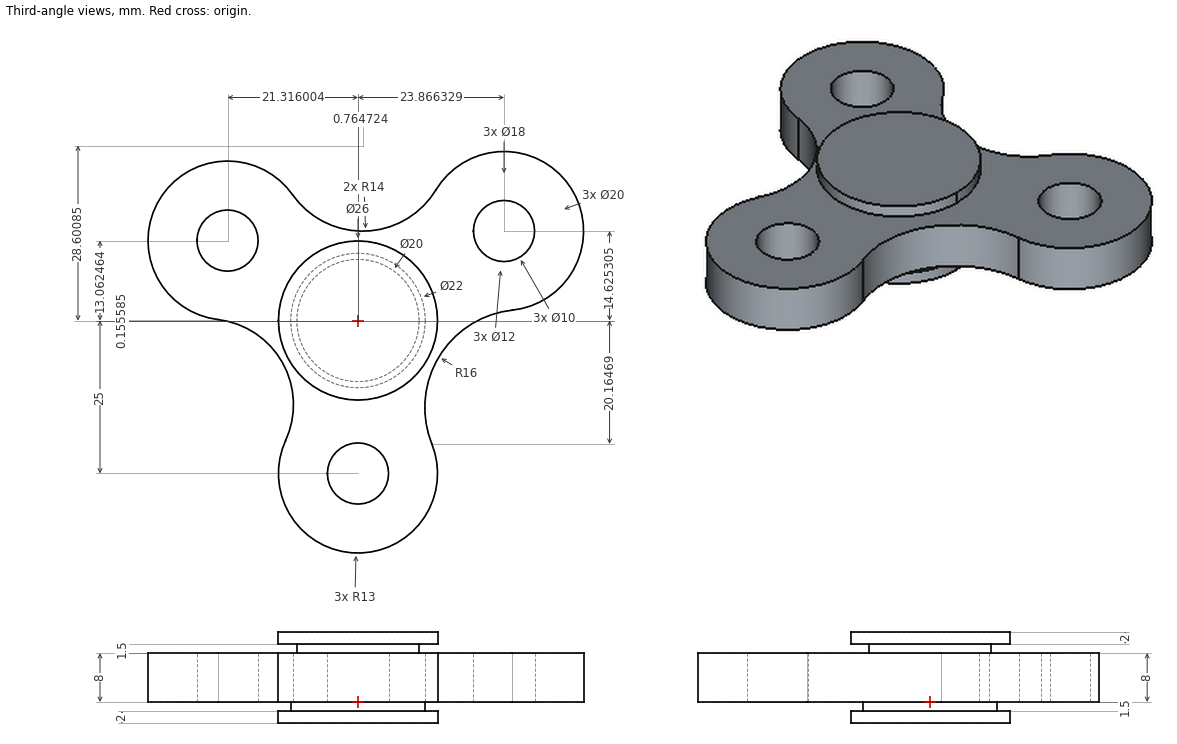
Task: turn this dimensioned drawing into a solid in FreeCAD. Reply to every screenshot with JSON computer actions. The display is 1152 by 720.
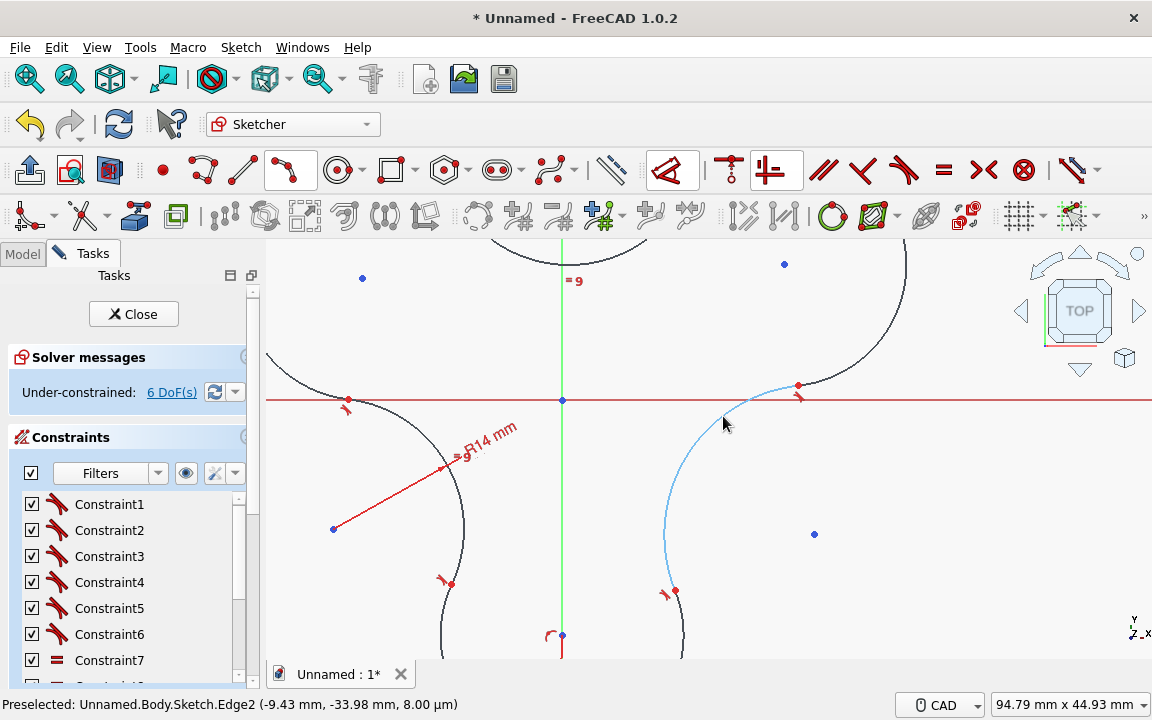
{"action": "left_click", "coordinate": [722, 416]}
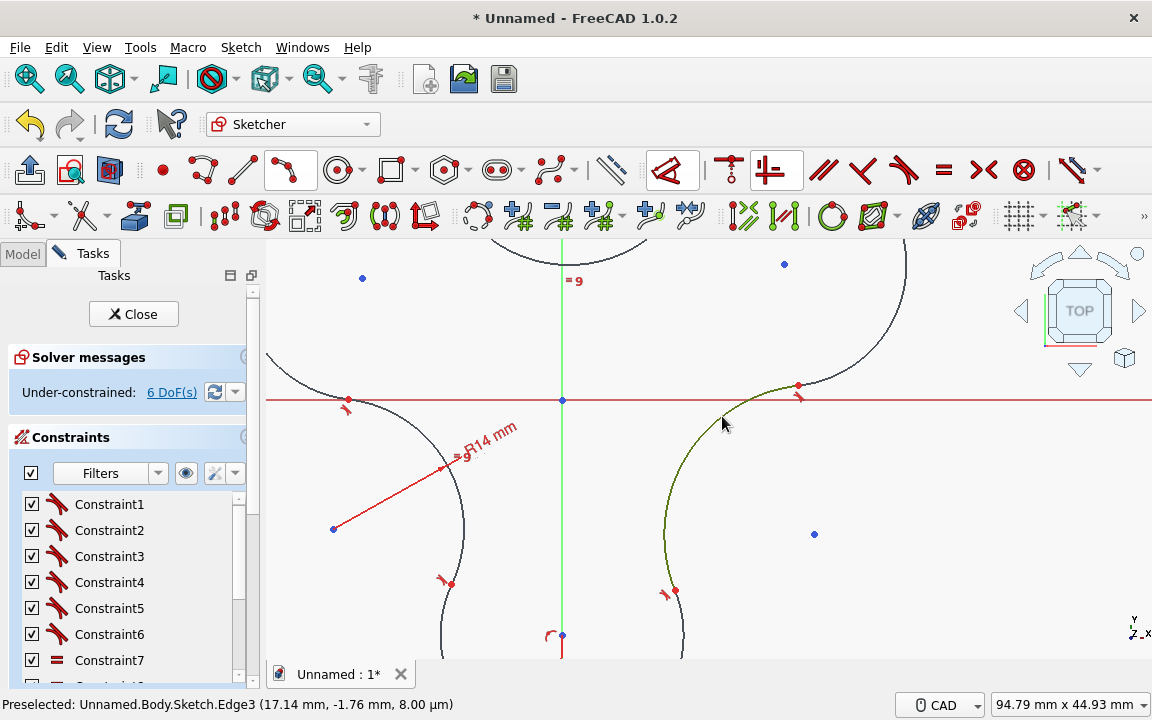
{"action": "left_click", "coordinate": [694, 170]}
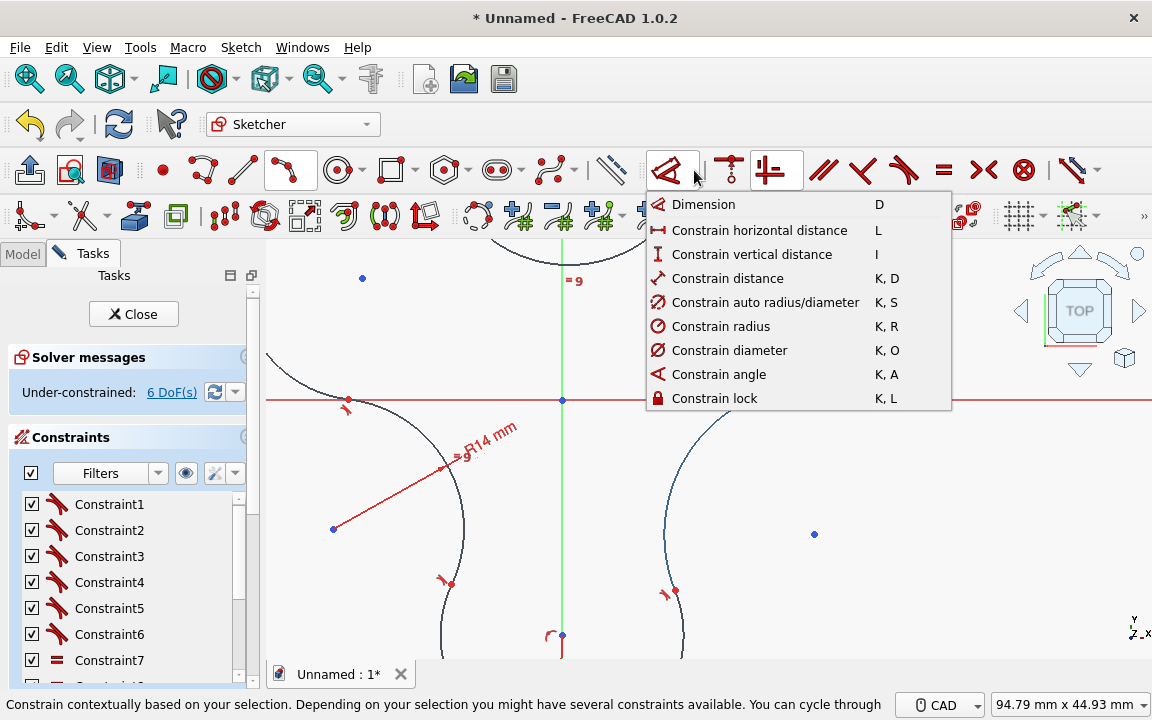
{"action": "left_click", "coordinate": [799, 326]}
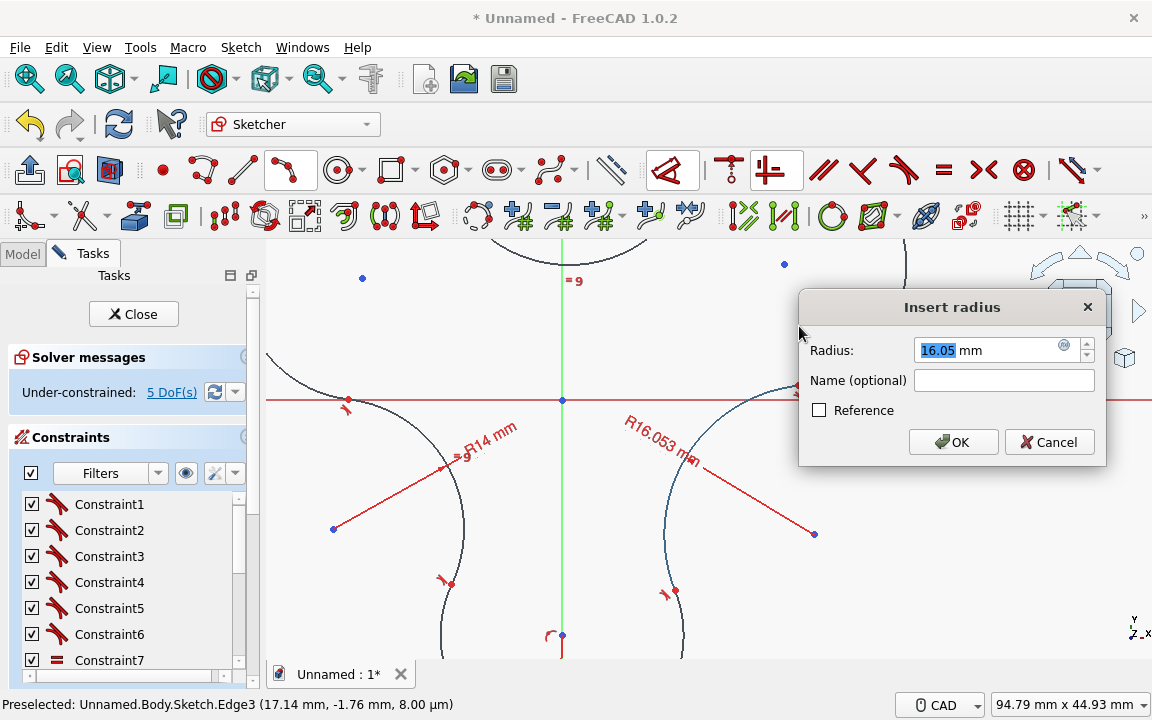
{"action": "type", "text": "16"}
{"action": "key", "text": "Return"}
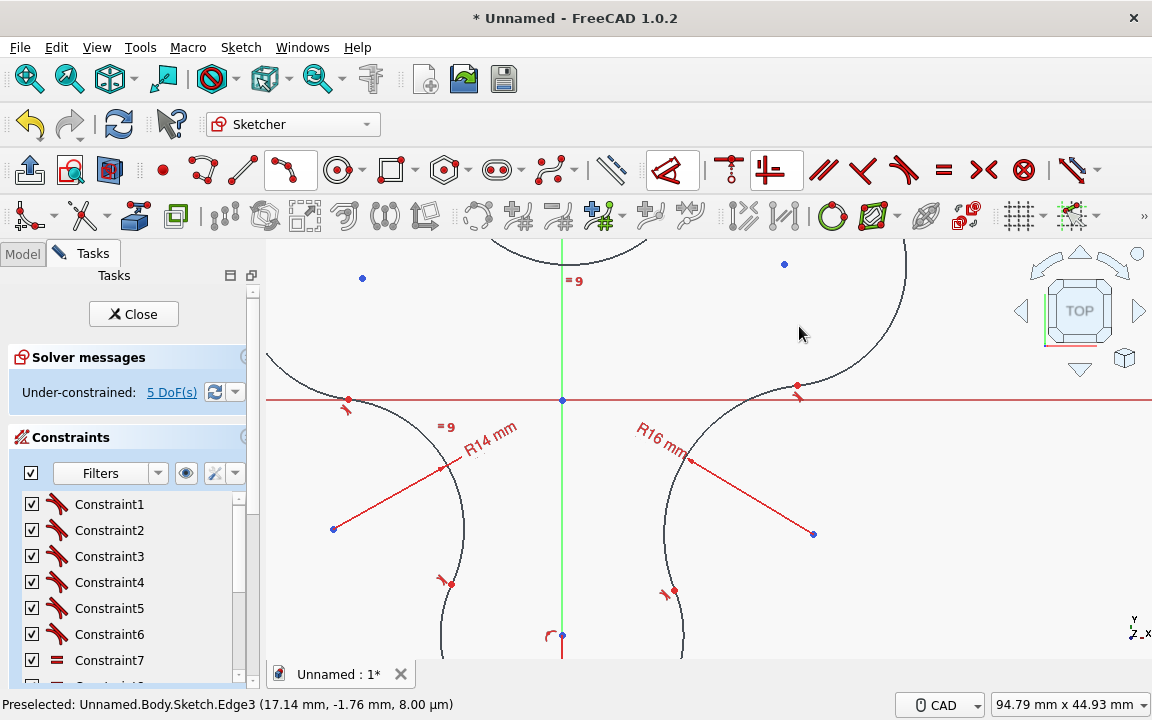
{"action": "scroll", "coordinate": [695, 426], "scroll_direction": "down", "scroll_amount": 4}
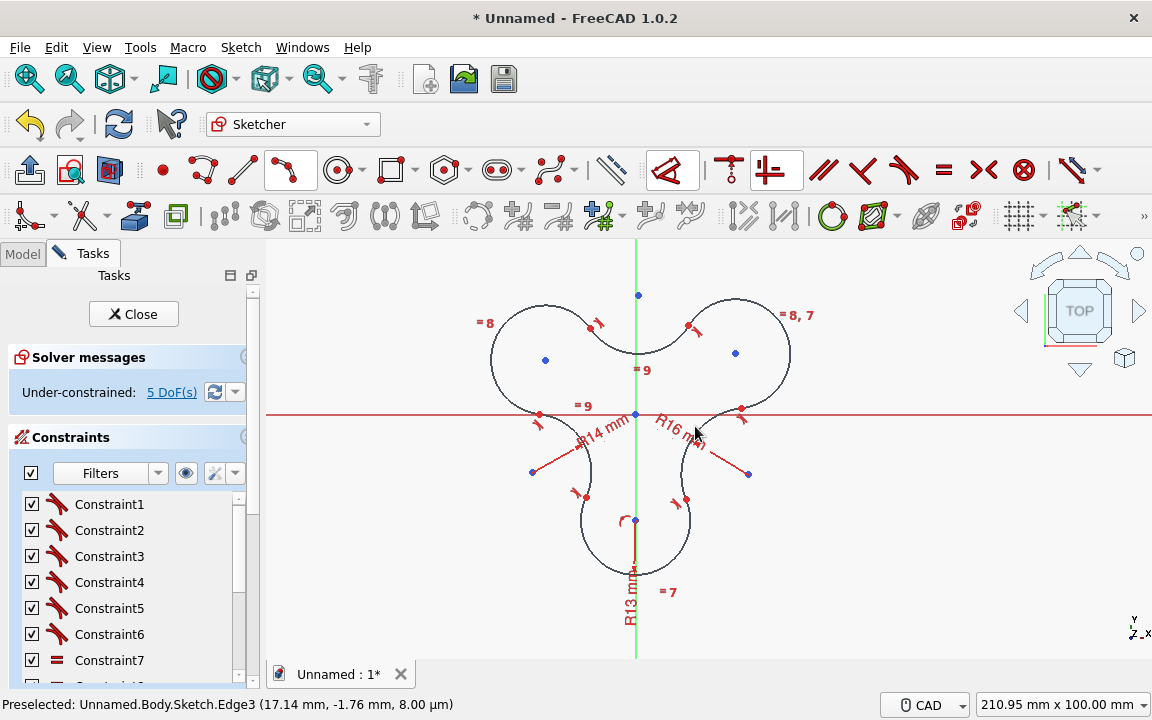
{"action": "left_click", "coordinate": [636, 520]}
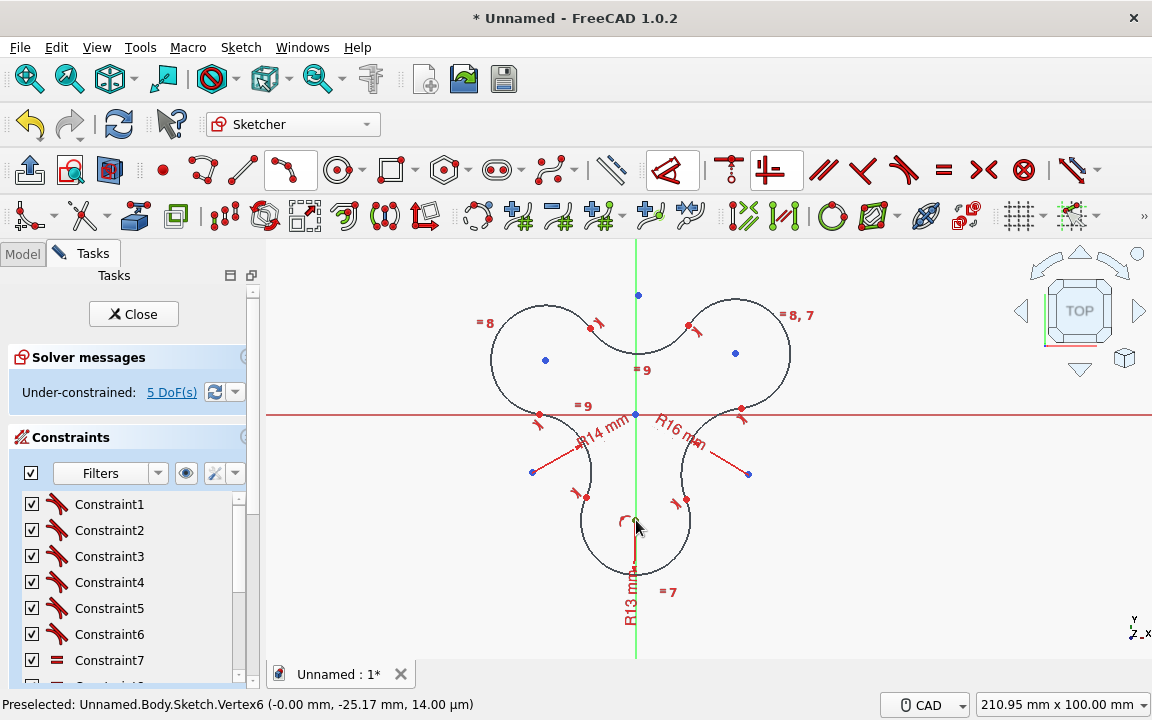
{"action": "left_click", "coordinate": [694, 170]}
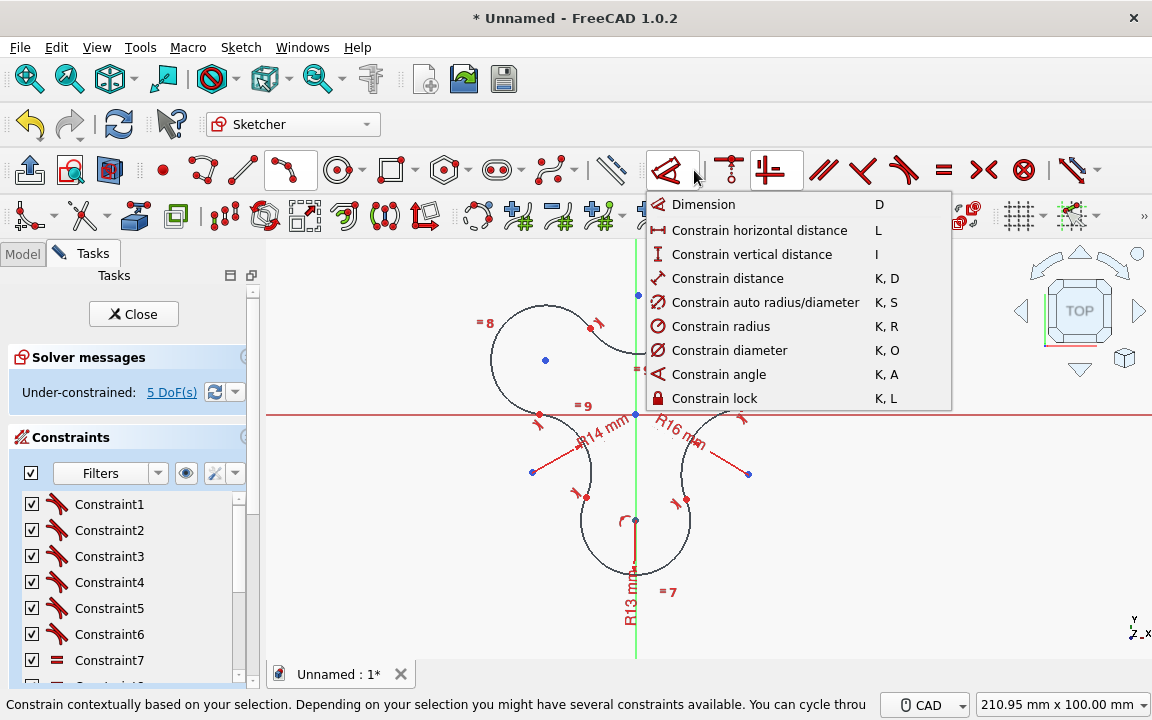
{"action": "left_click", "coordinate": [799, 254]}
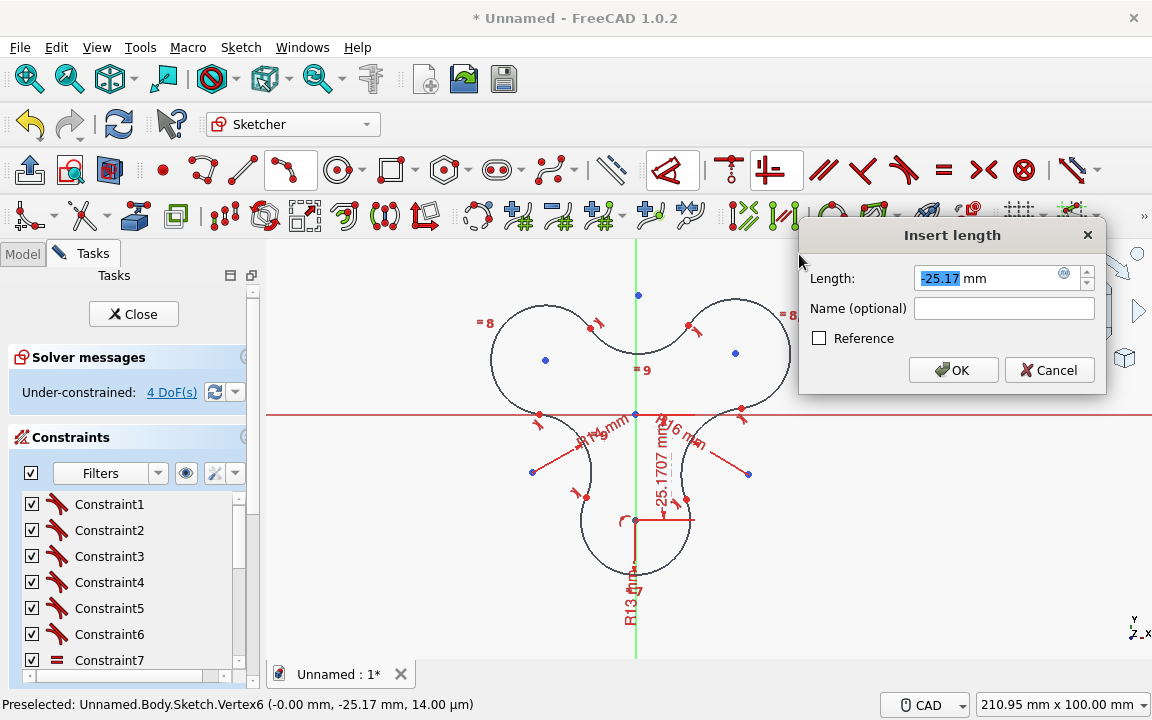
{"action": "type", "text": "-25"}
{"action": "key", "text": "Return"}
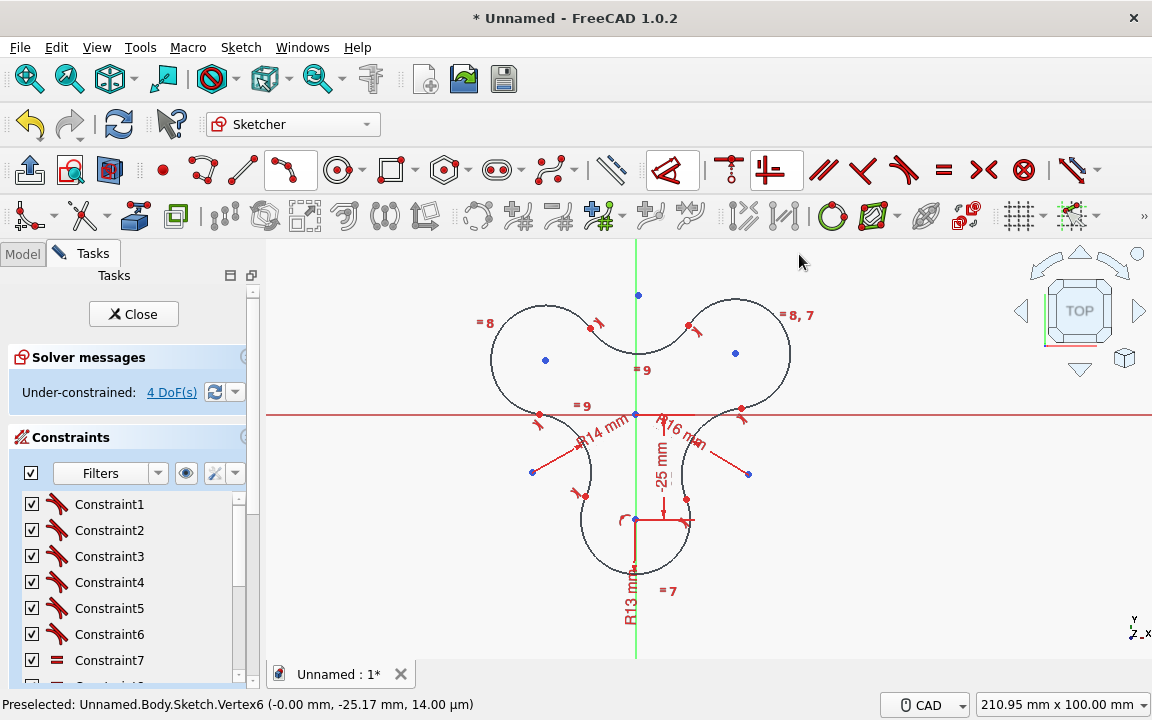
{"action": "scroll", "coordinate": [539, 414], "scroll_direction": "up", "scroll_amount": 21}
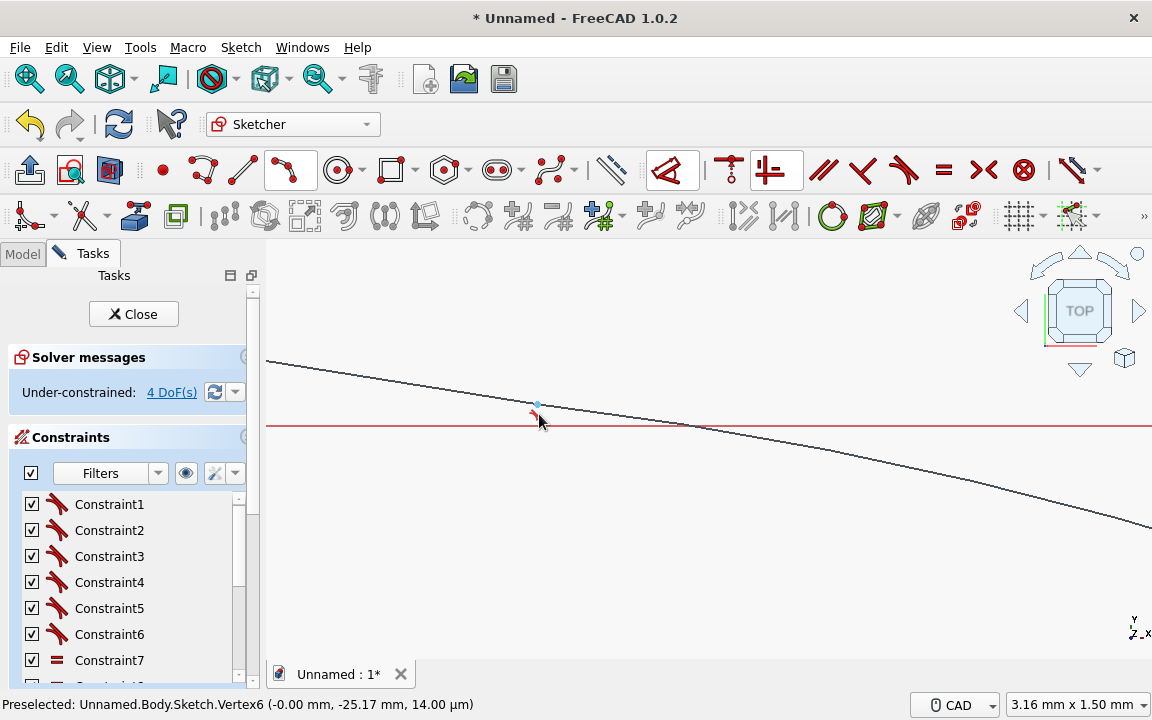
{"action": "left_click", "coordinate": [537, 404]}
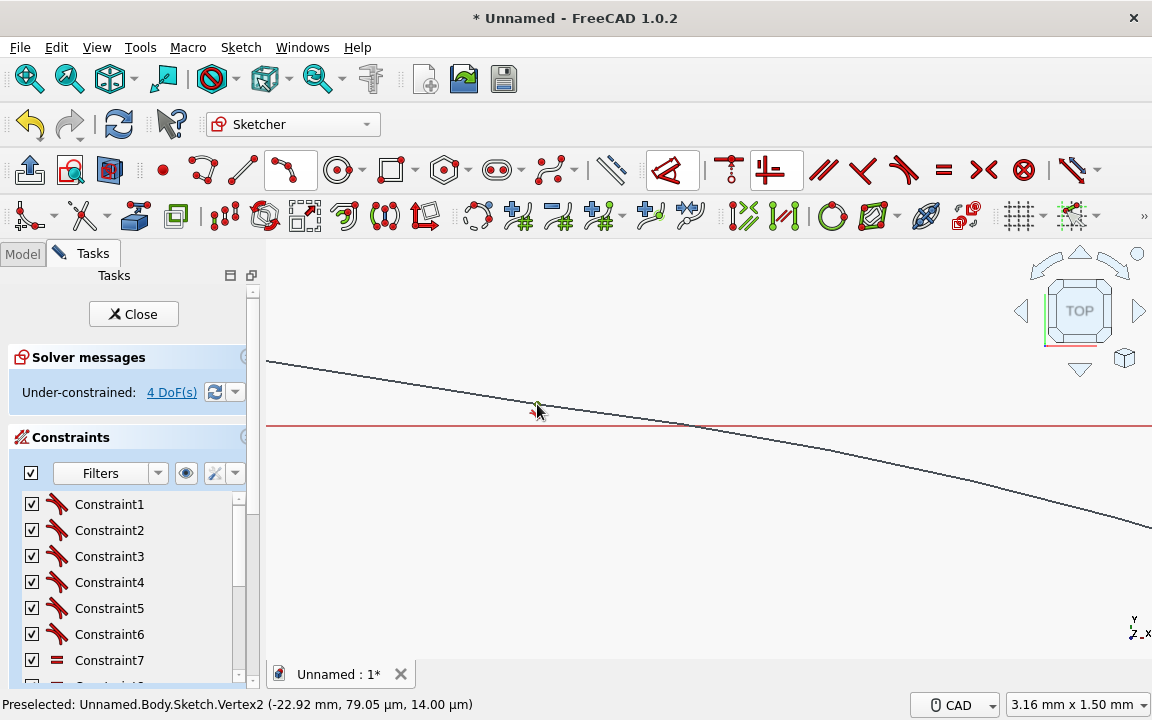
{"action": "left_click", "coordinate": [694, 170]}